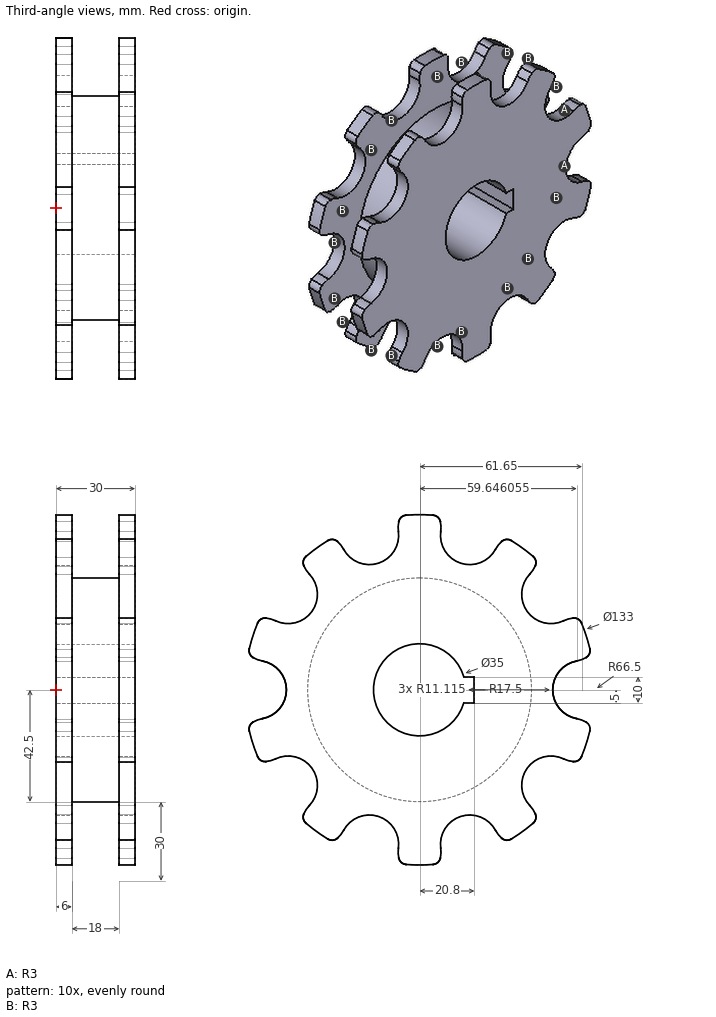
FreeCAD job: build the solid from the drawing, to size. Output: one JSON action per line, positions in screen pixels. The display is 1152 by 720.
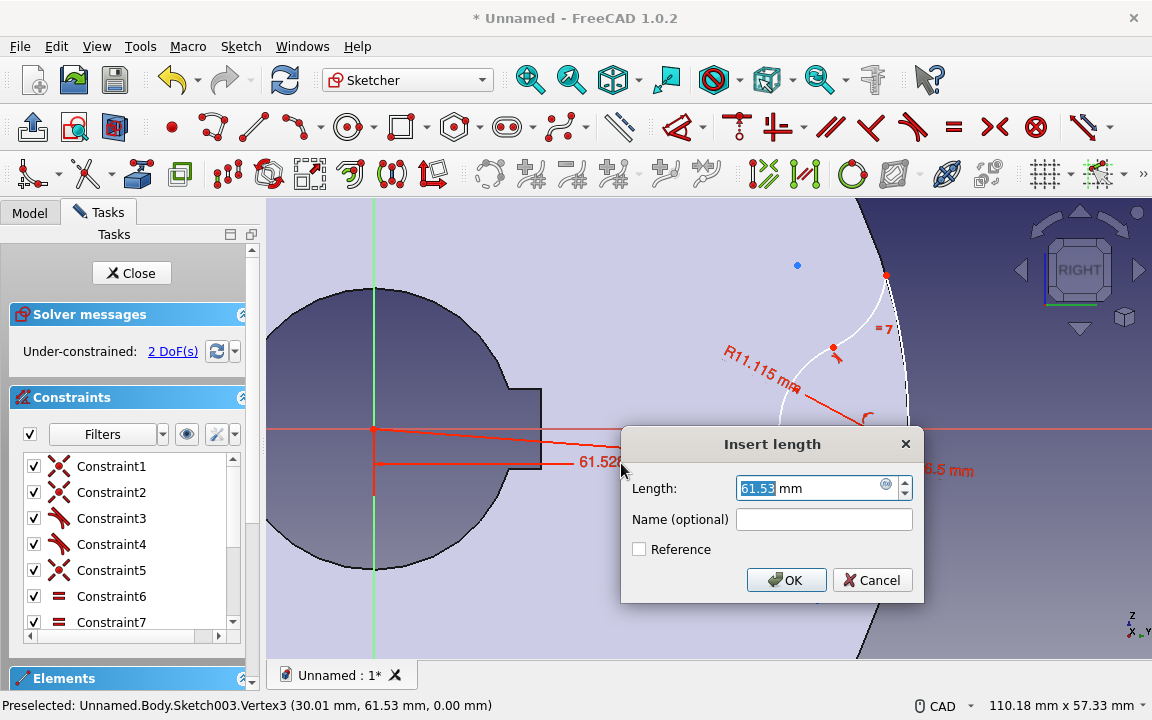
{"action": "type", "text": "61.65"}
{"action": "key", "text": "Return"}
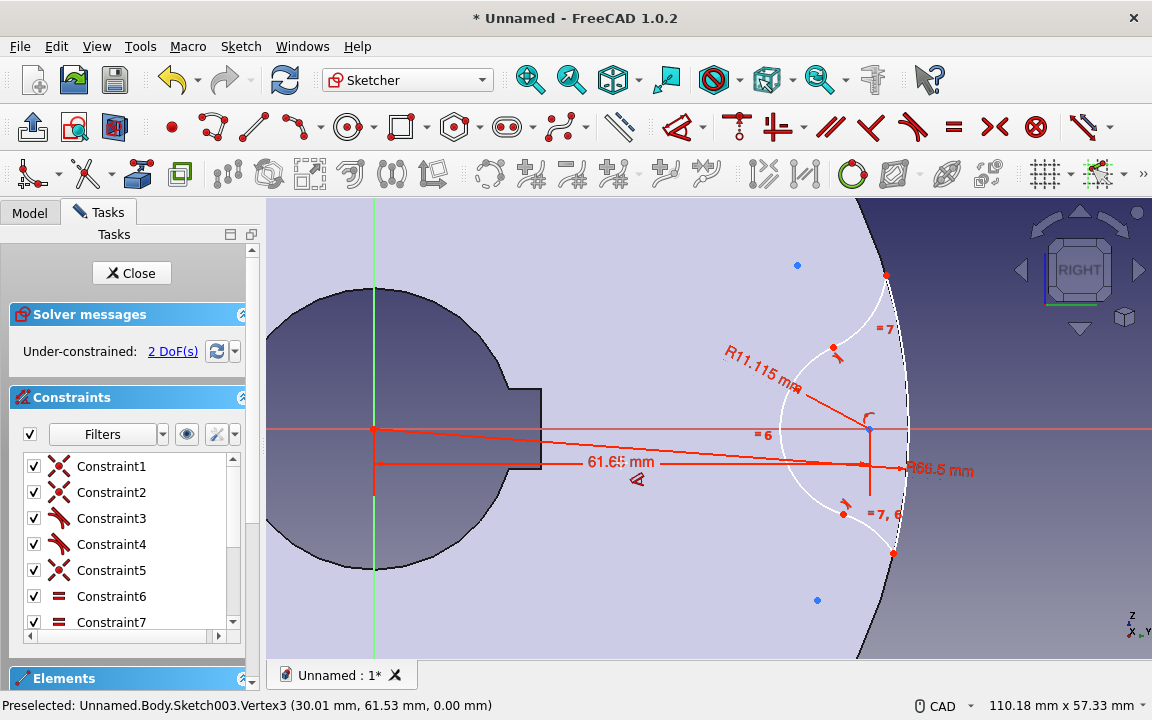
{"action": "left_click", "coordinate": [834, 347]}
{"action": "left_click", "coordinate": [604, 313]}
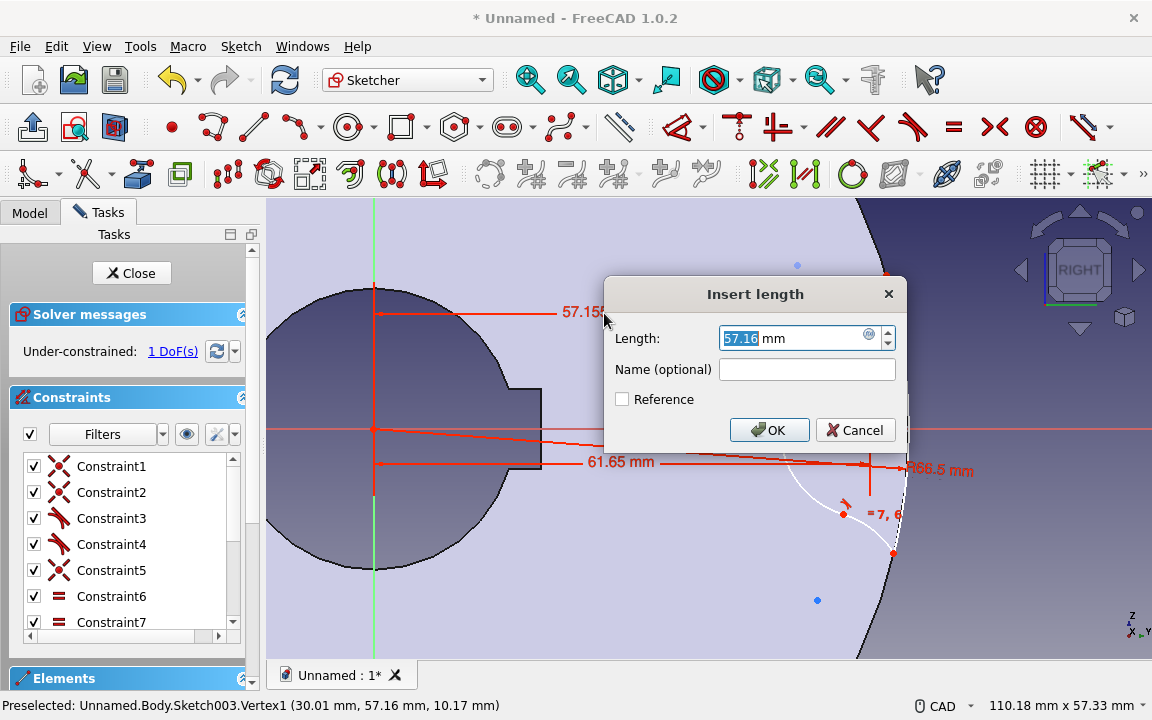
{"action": "type", "text": "59.646055"}
{"action": "key", "text": "Return"}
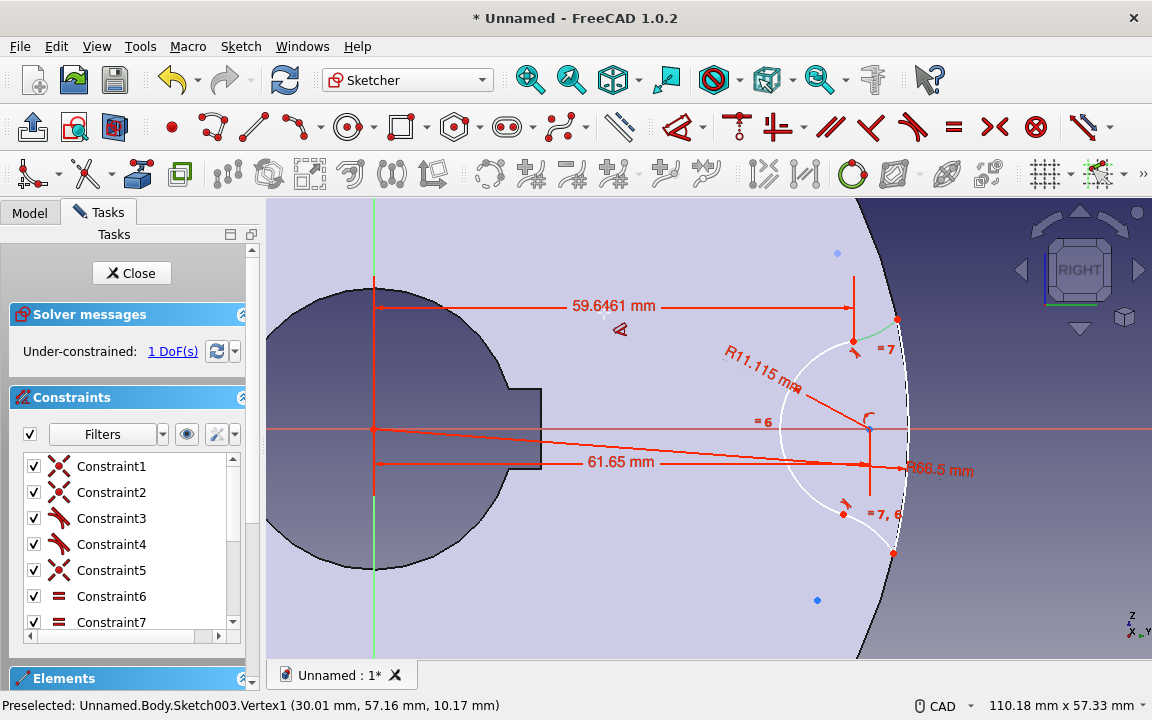
{"action": "left_click", "coordinate": [844, 515]}
{"action": "left_click", "coordinate": [609, 549]}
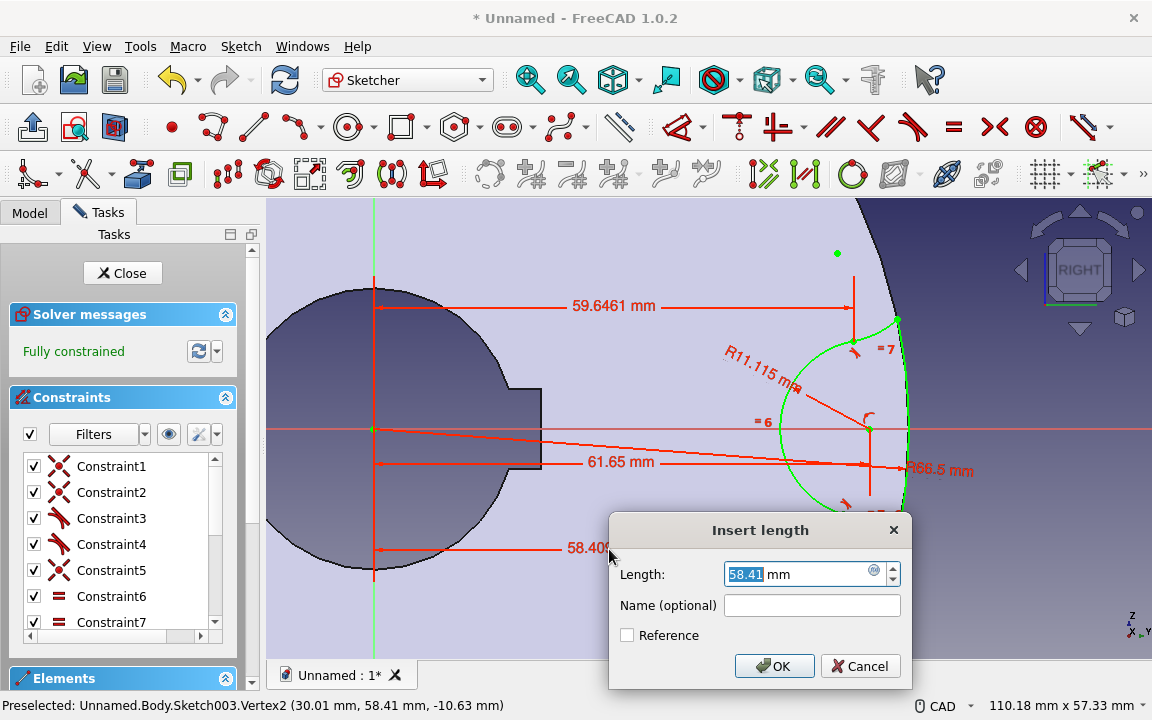
{"action": "type", "text": "59.646055"}
{"action": "key", "text": "Return"}
{"action": "key", "text": "Escape"}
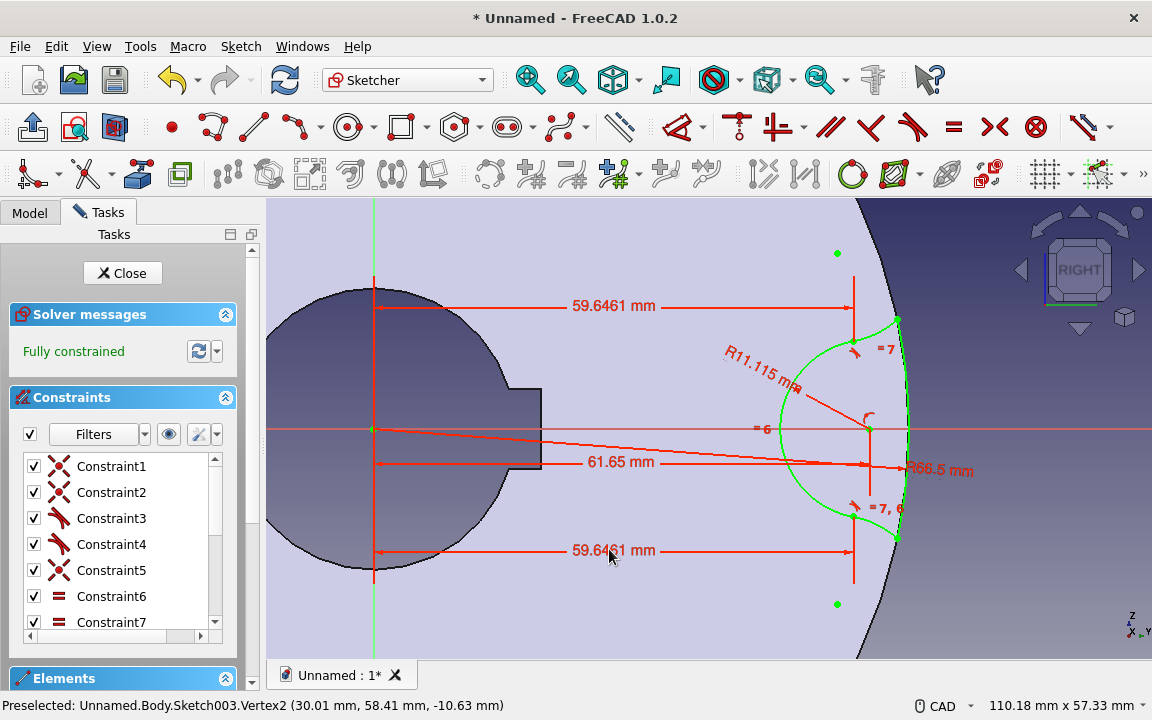
{"action": "left_click", "coordinate": [123, 273]}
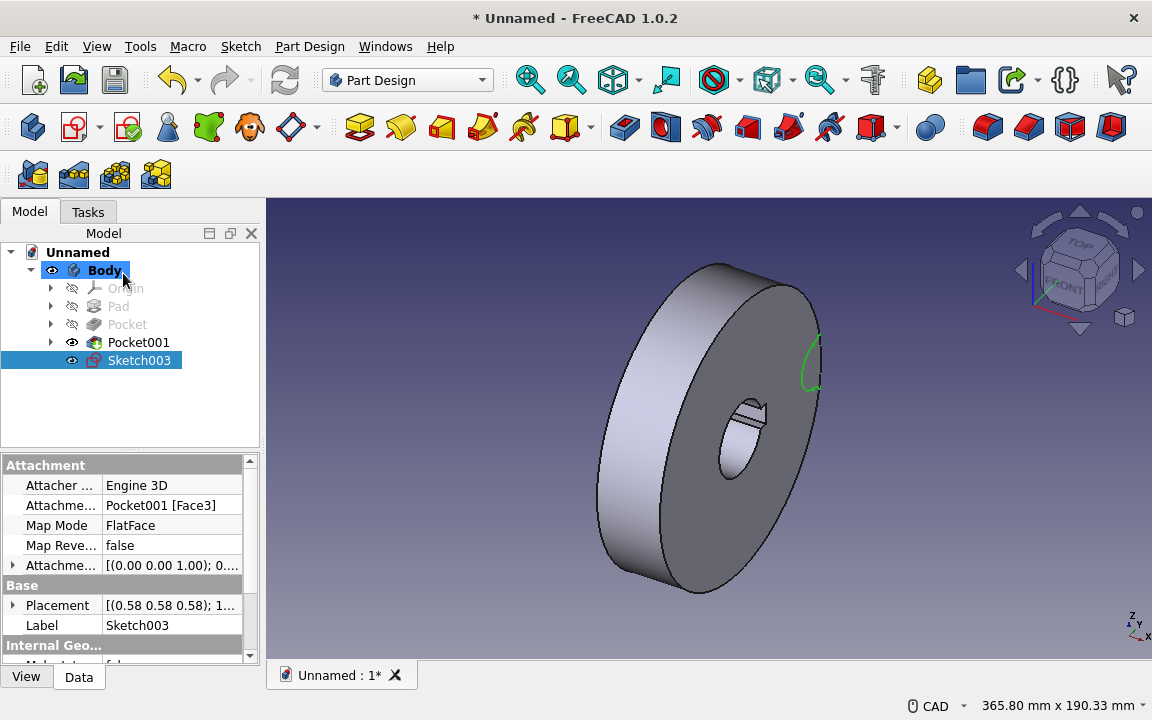
{"action": "left_click", "coordinate": [625, 128]}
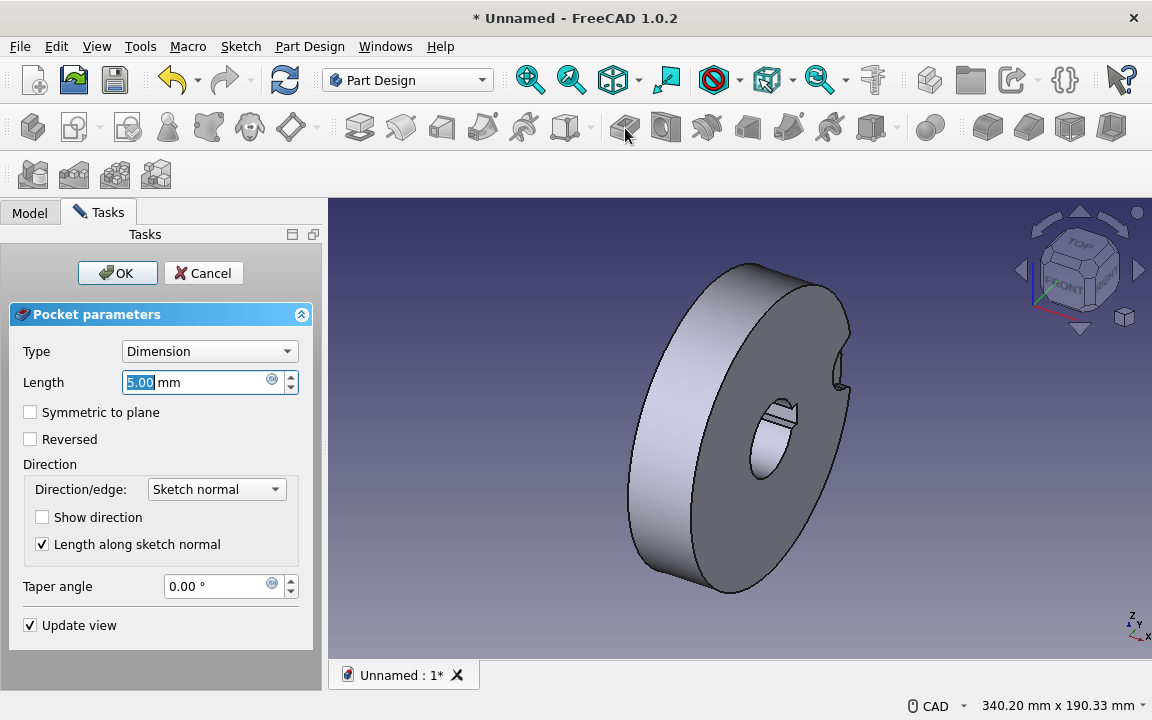
{"action": "left_click", "coordinate": [210, 352]}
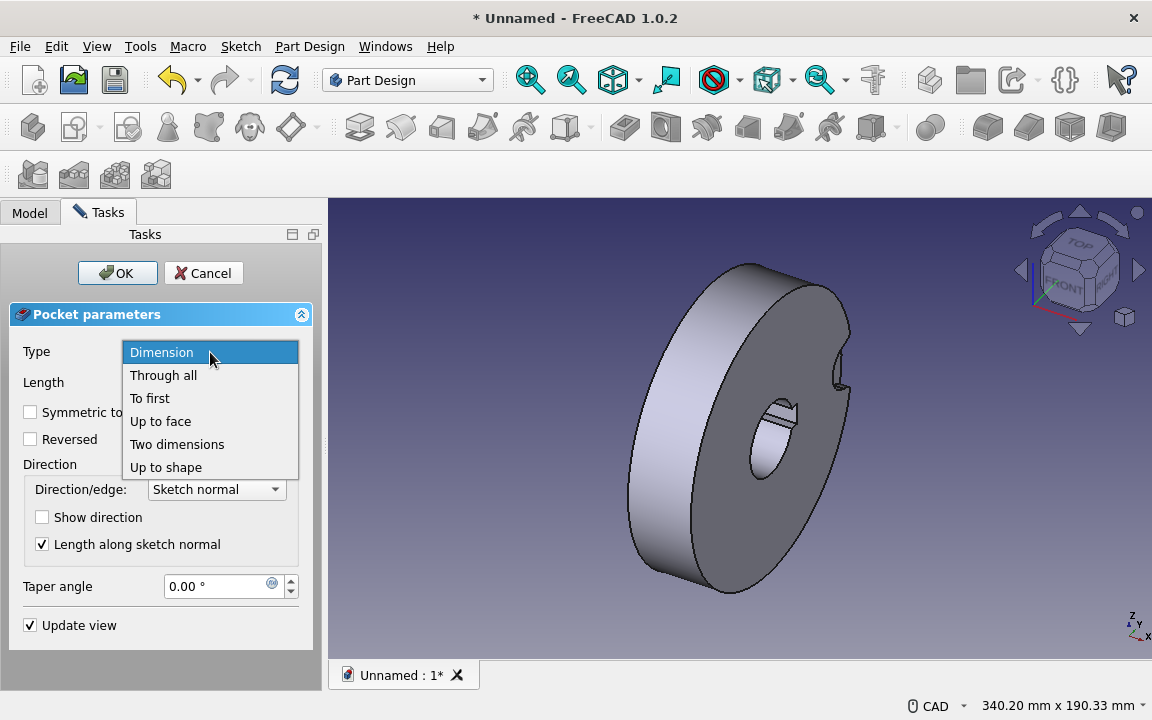
{"action": "left_click", "coordinate": [208, 376]}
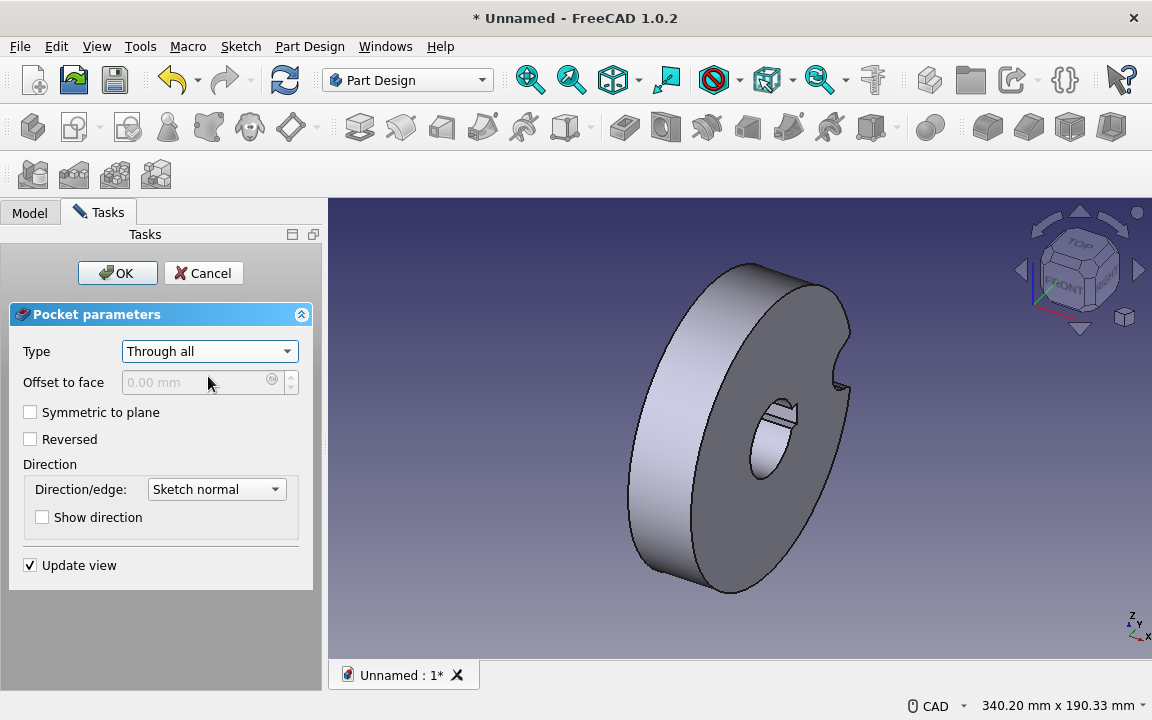
{"action": "left_click", "coordinate": [118, 273]}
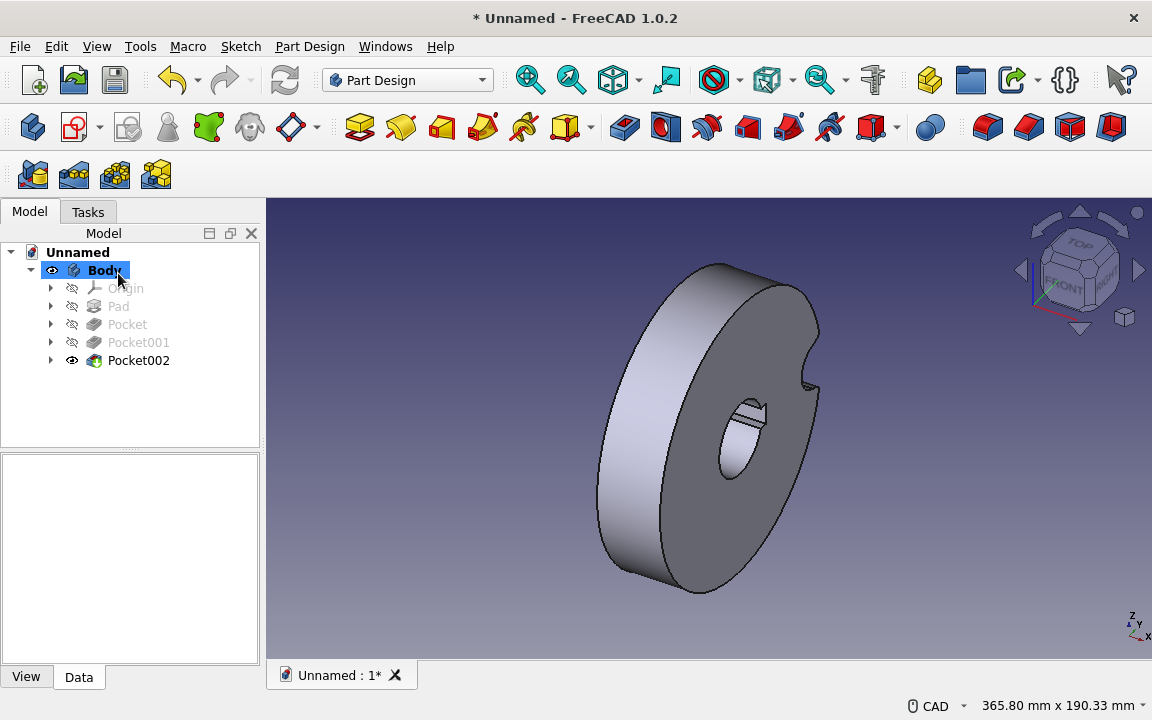
{"action": "key", "text": "0"}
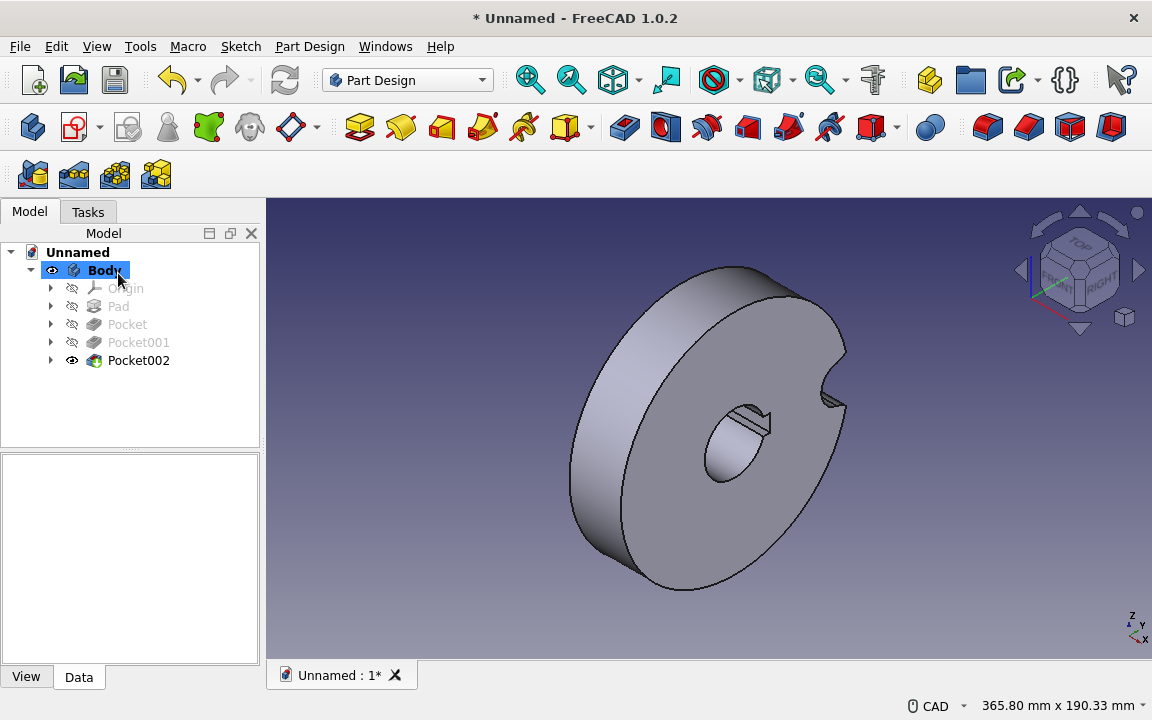
{"action": "key", "text": "2"}